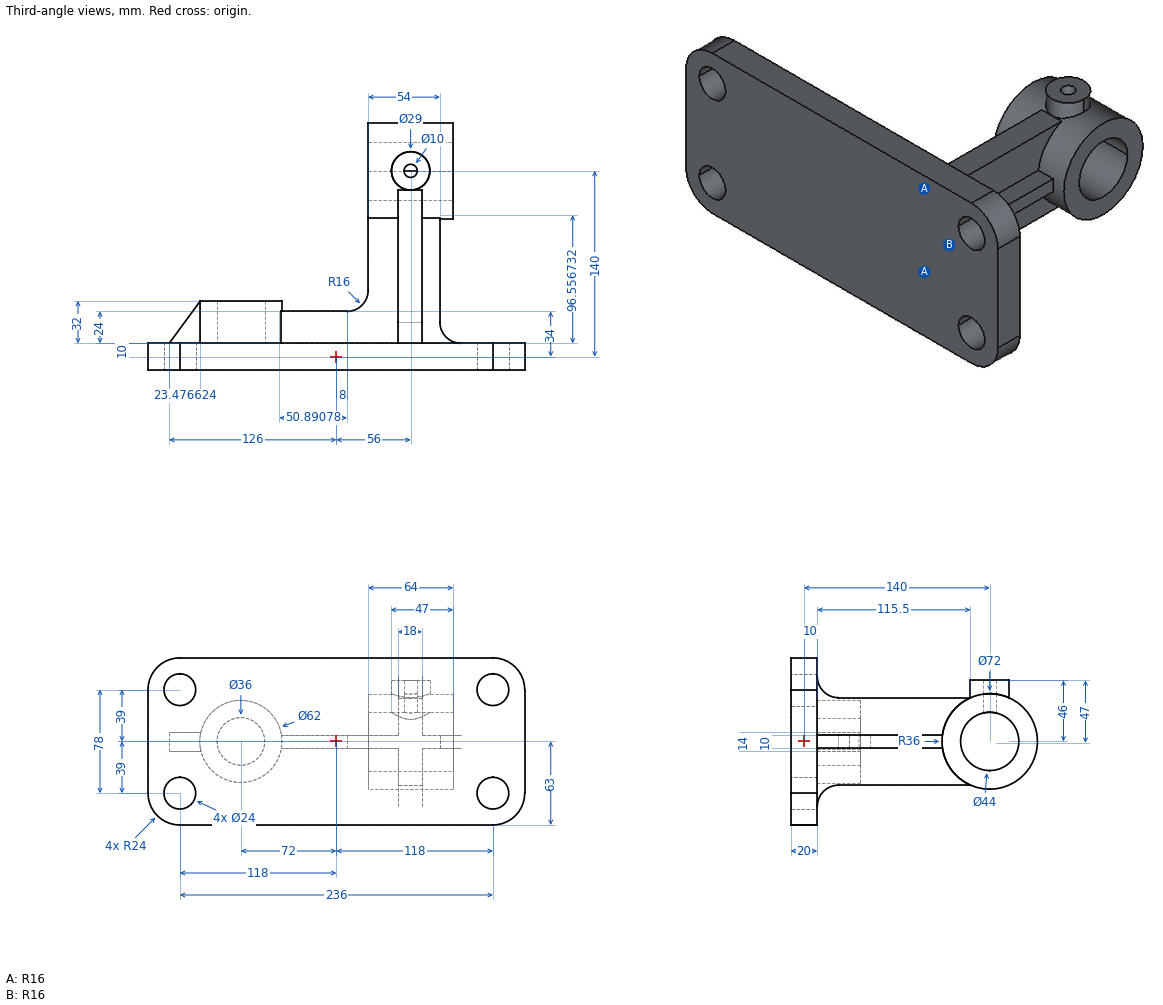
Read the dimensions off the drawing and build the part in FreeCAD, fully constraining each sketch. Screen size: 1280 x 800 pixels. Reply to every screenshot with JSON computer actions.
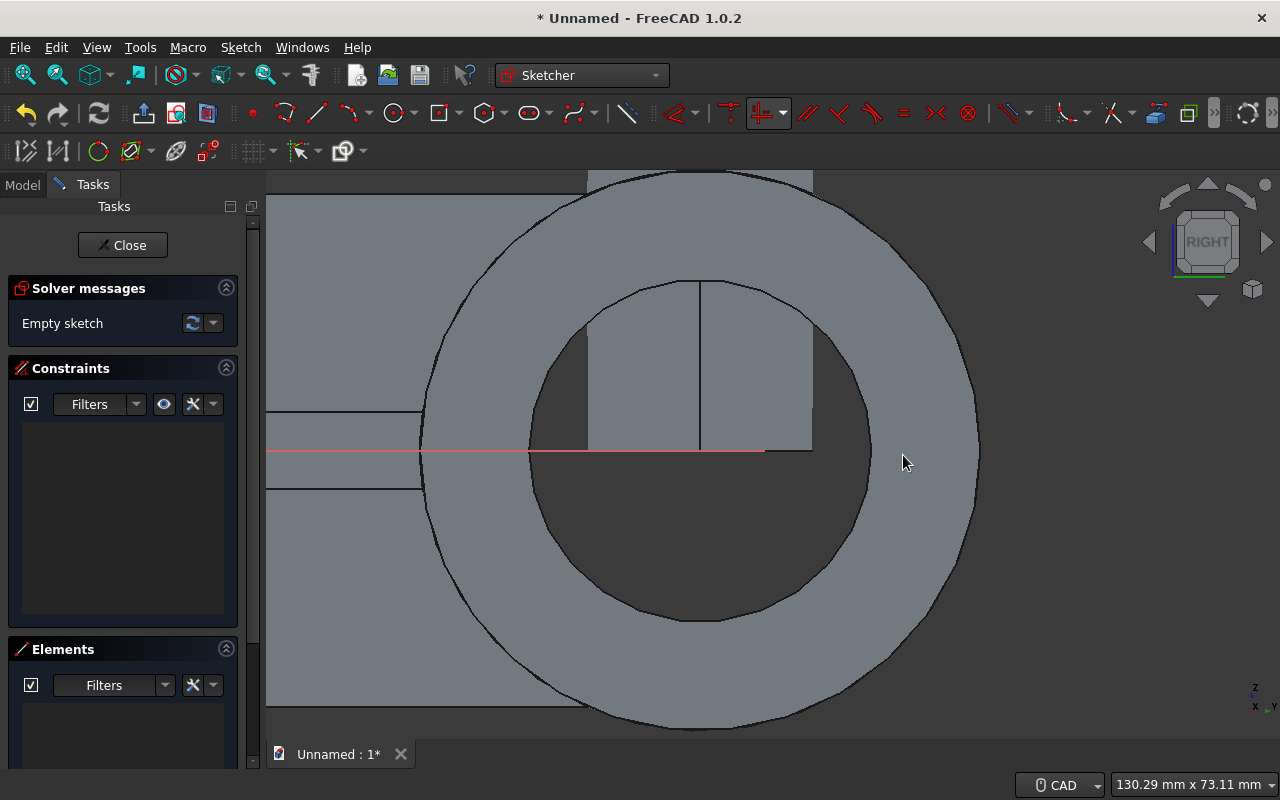
{"action": "left_click", "coordinate": [394, 114]}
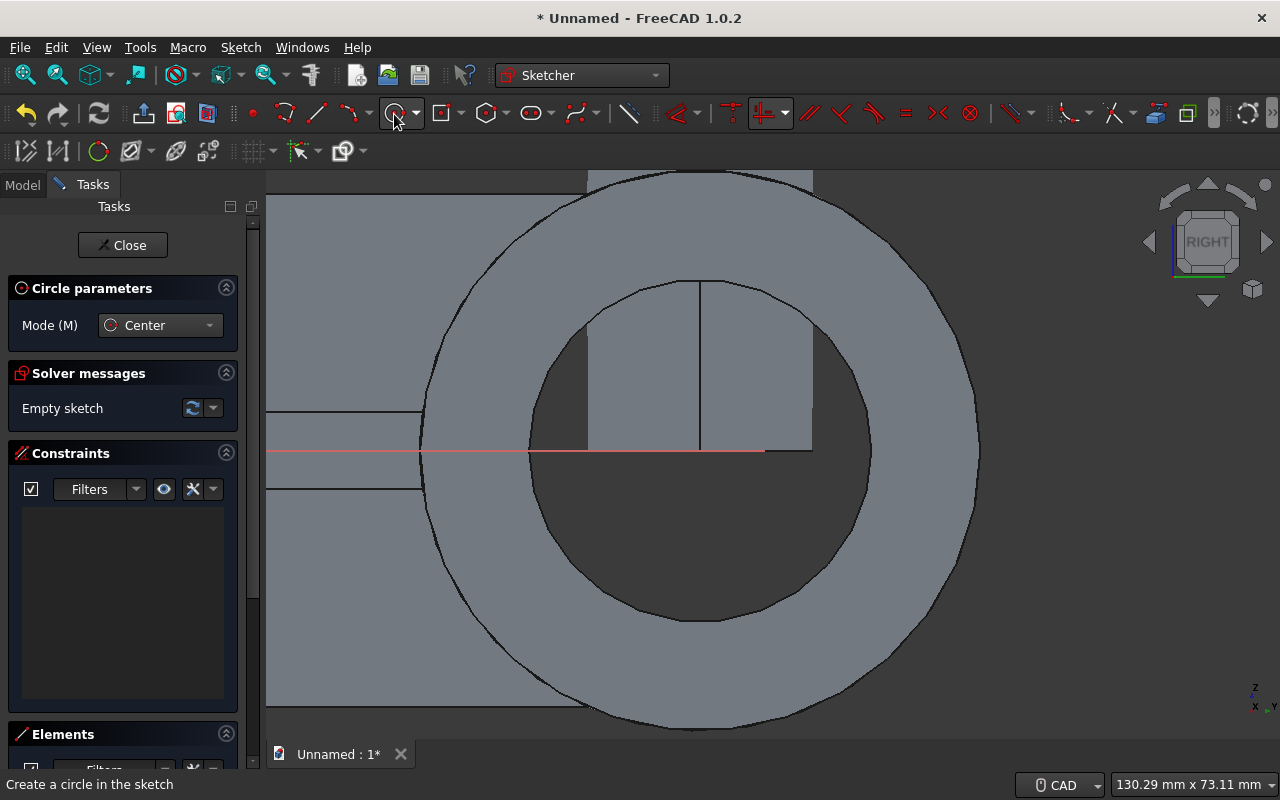
{"action": "left_click", "coordinate": [700, 451]}
{"action": "mouse_move", "coordinate": [821, 329]}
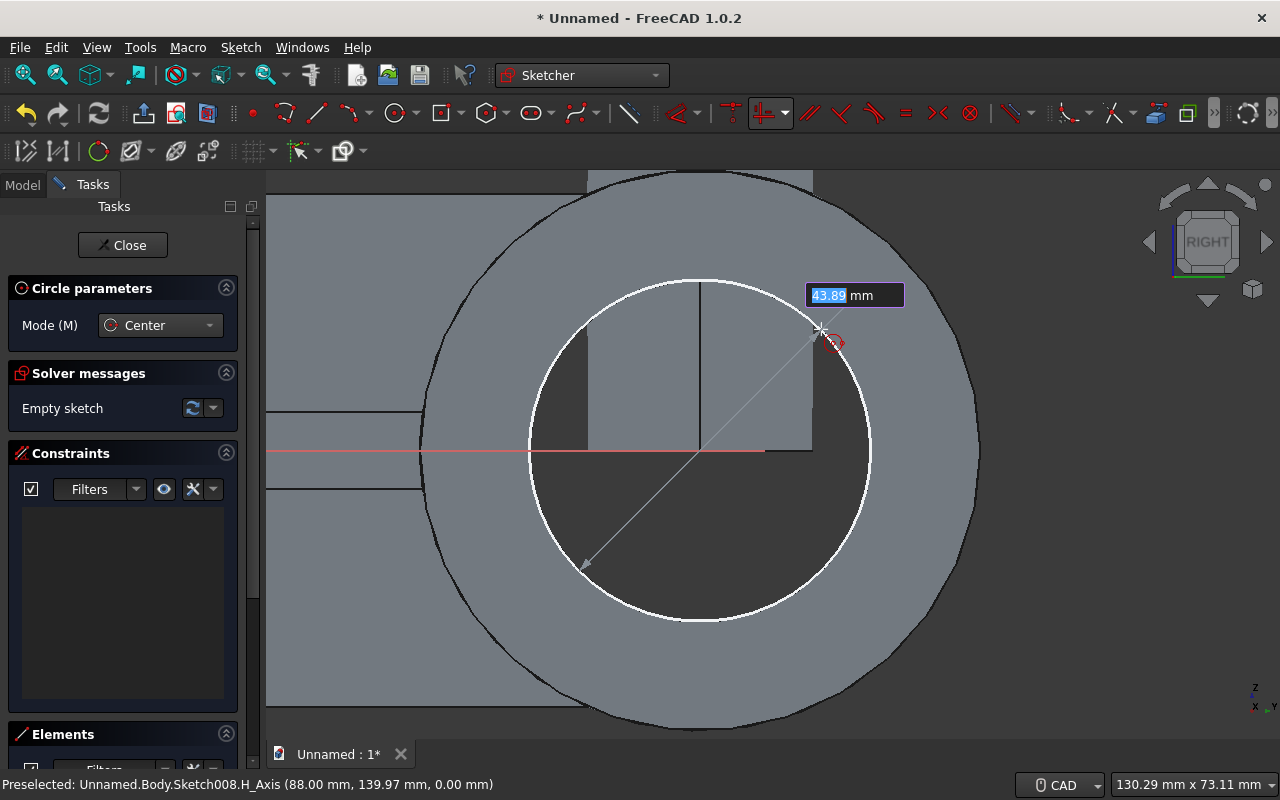
{"action": "type", "text": "44"}
{"action": "key", "text": "Return"}
{"action": "key", "text": "Escape"}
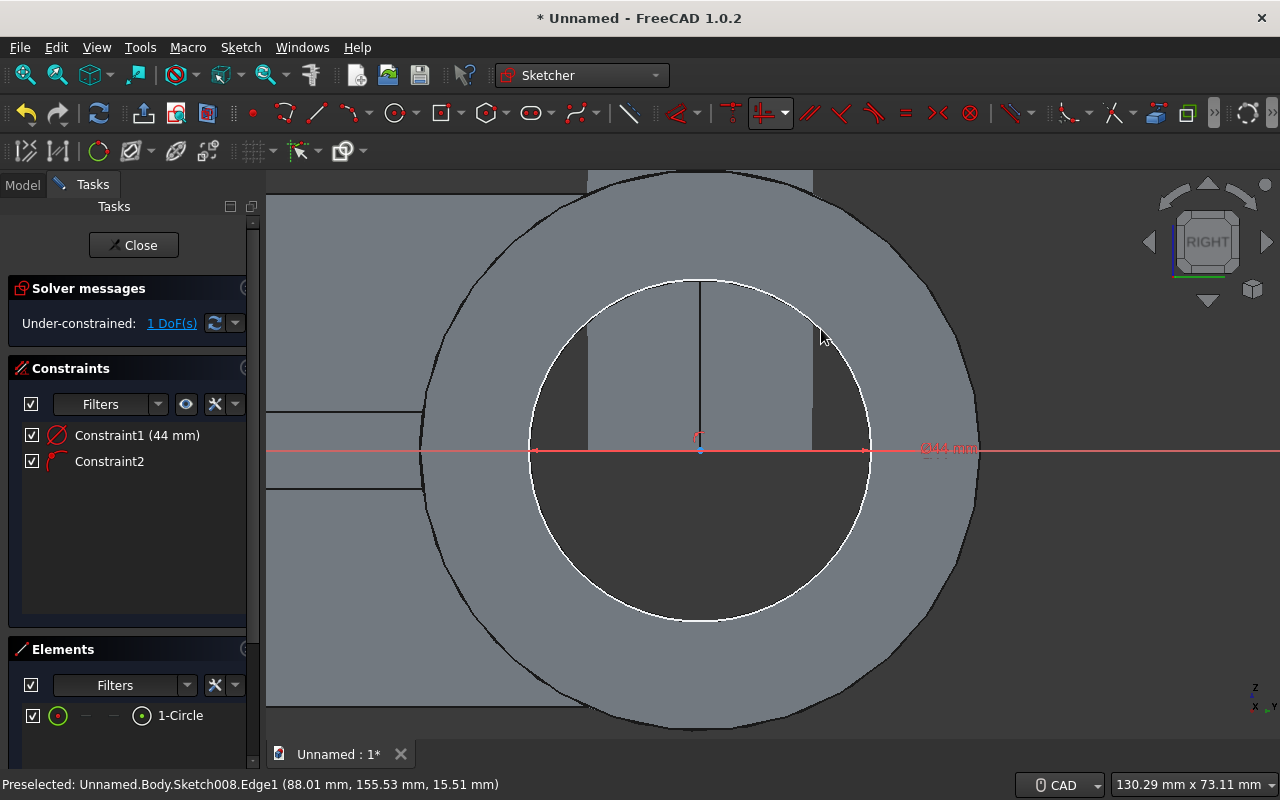
{"action": "left_click", "coordinate": [676, 114]}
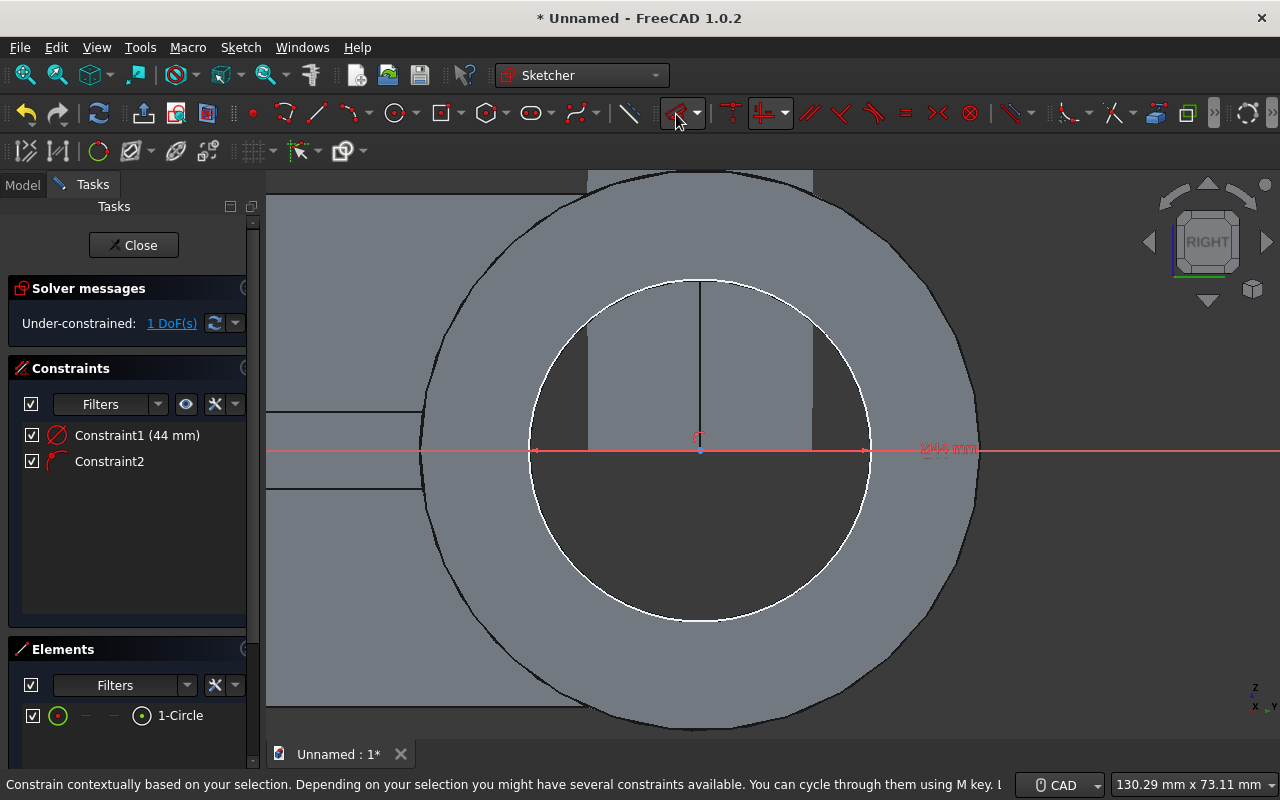
{"action": "left_click", "coordinate": [700, 451]}
{"action": "left_click", "coordinate": [497, 485]}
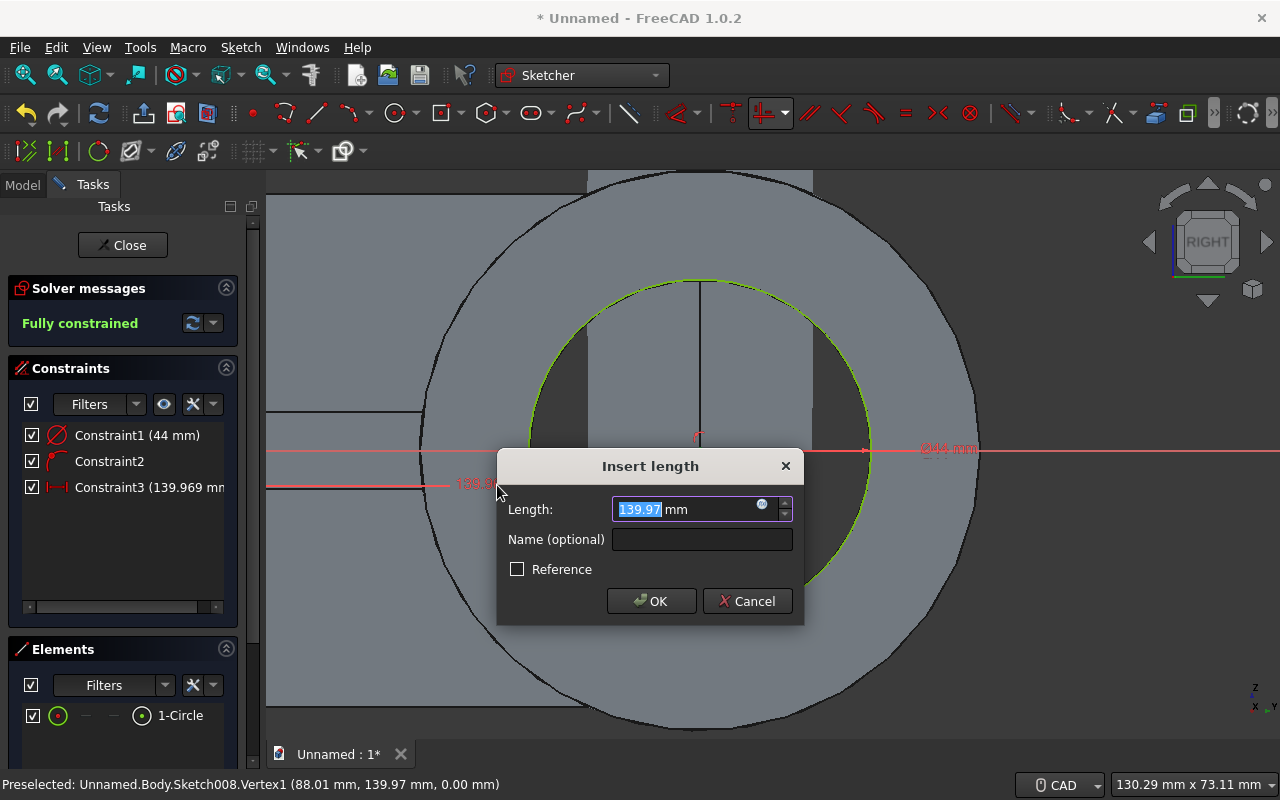
{"action": "type", "text": "140"}
{"action": "key", "text": "Return"}
{"action": "key", "text": "Escape"}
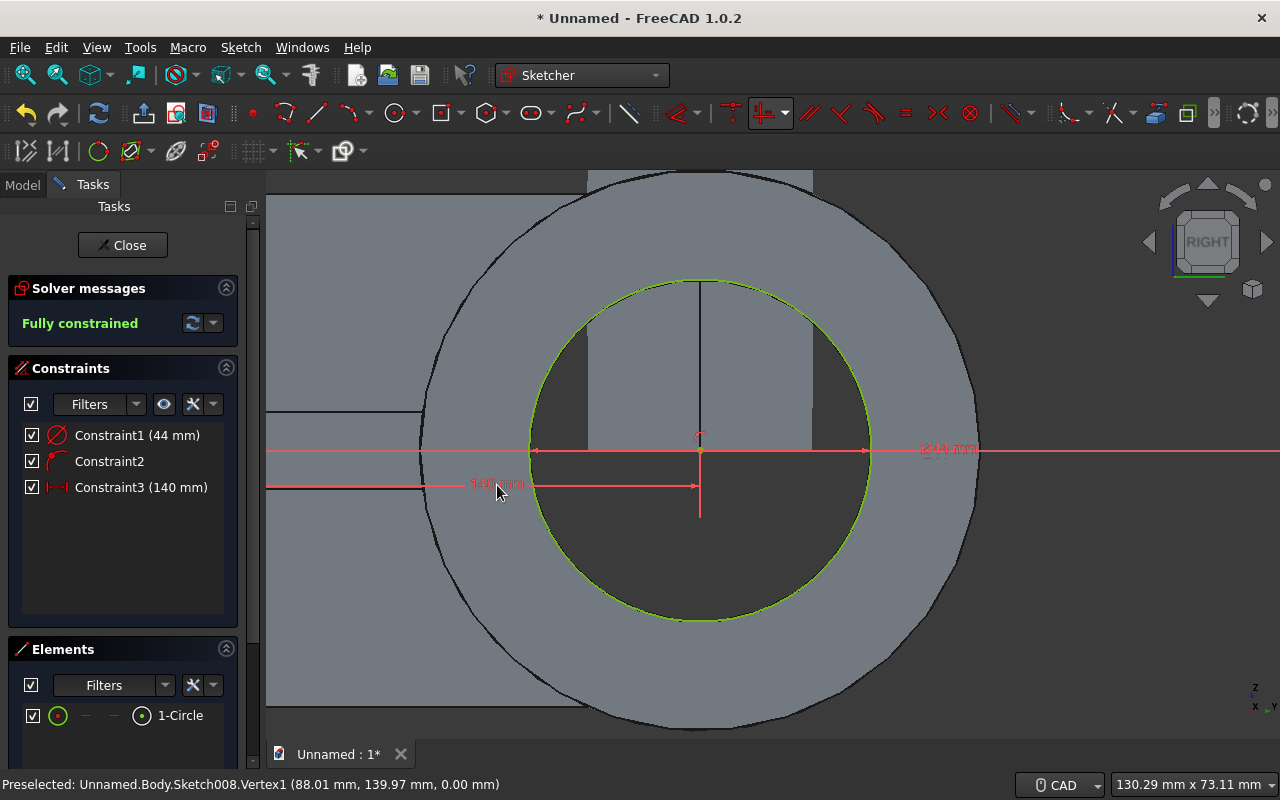
{"action": "left_click", "coordinate": [123, 245]}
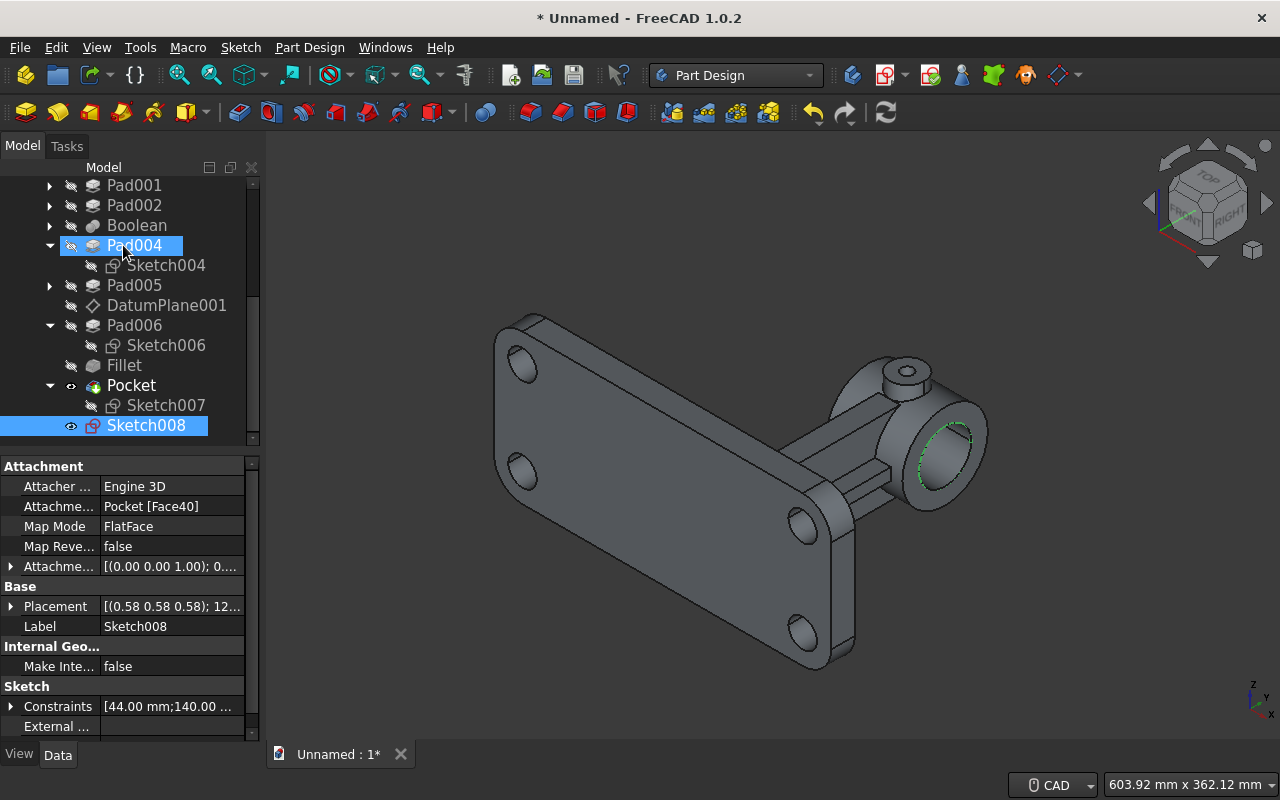
{"action": "left_click", "coordinate": [240, 112]}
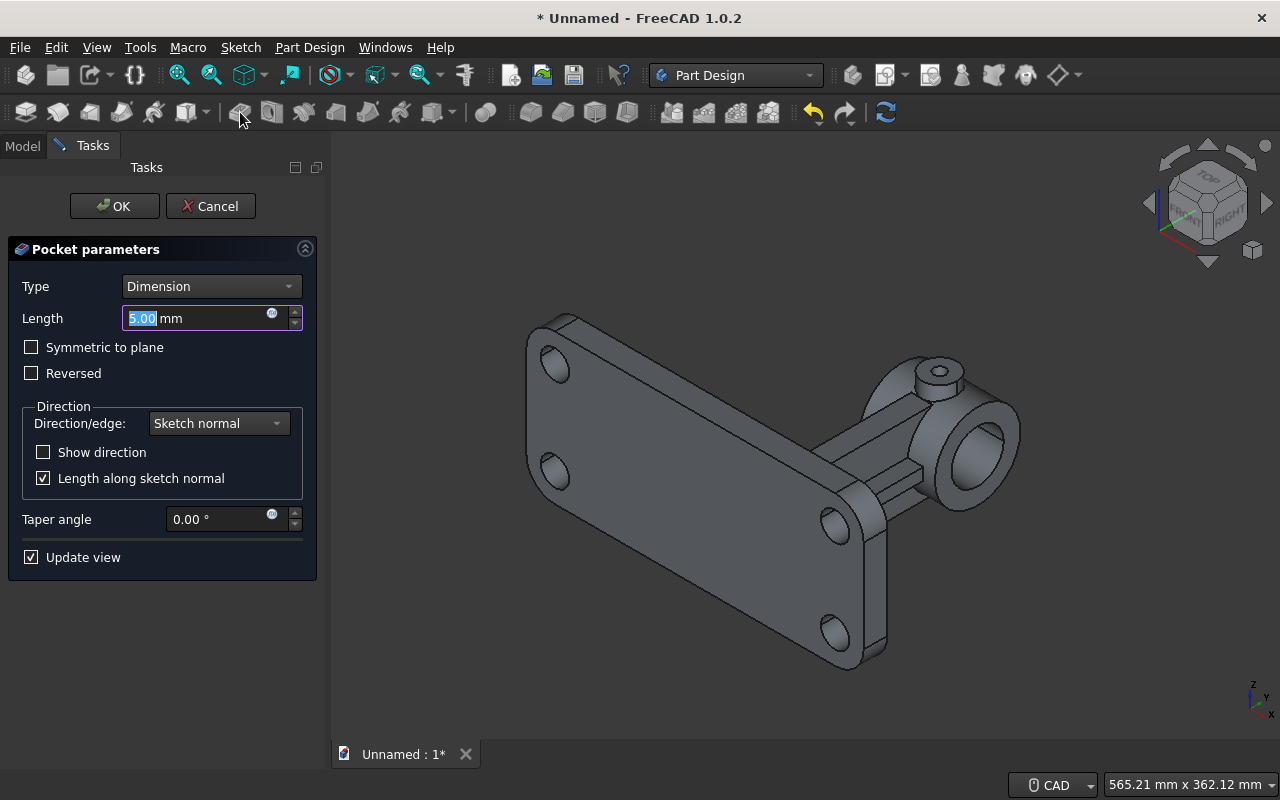
{"action": "type", "text": "47"}
{"action": "key", "text": "Tab"}